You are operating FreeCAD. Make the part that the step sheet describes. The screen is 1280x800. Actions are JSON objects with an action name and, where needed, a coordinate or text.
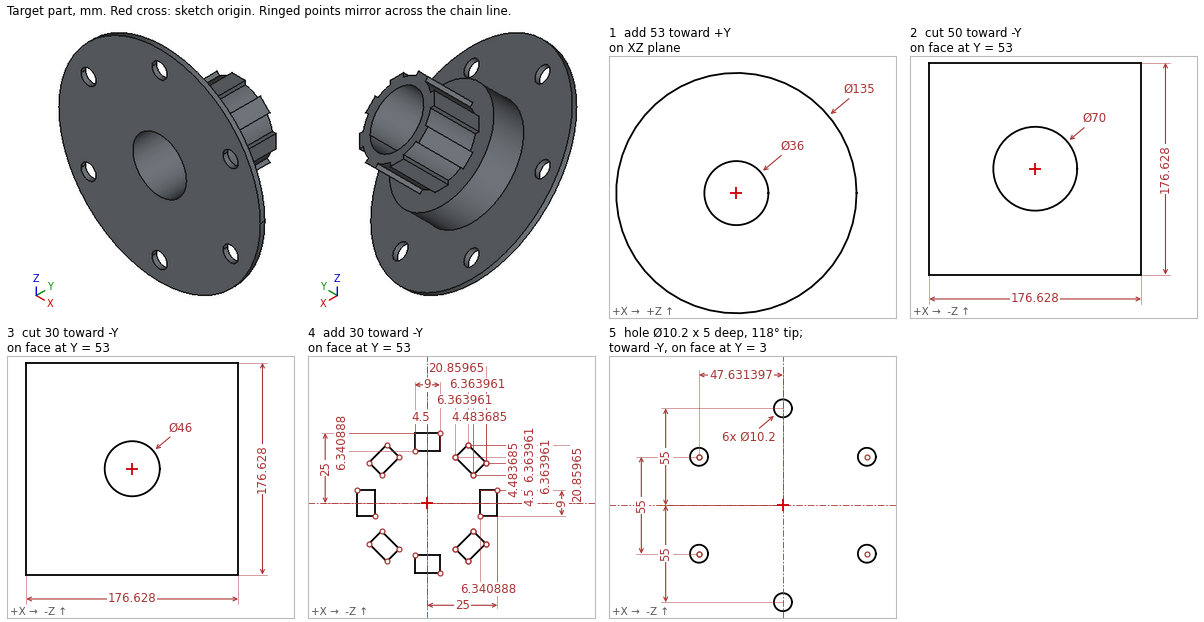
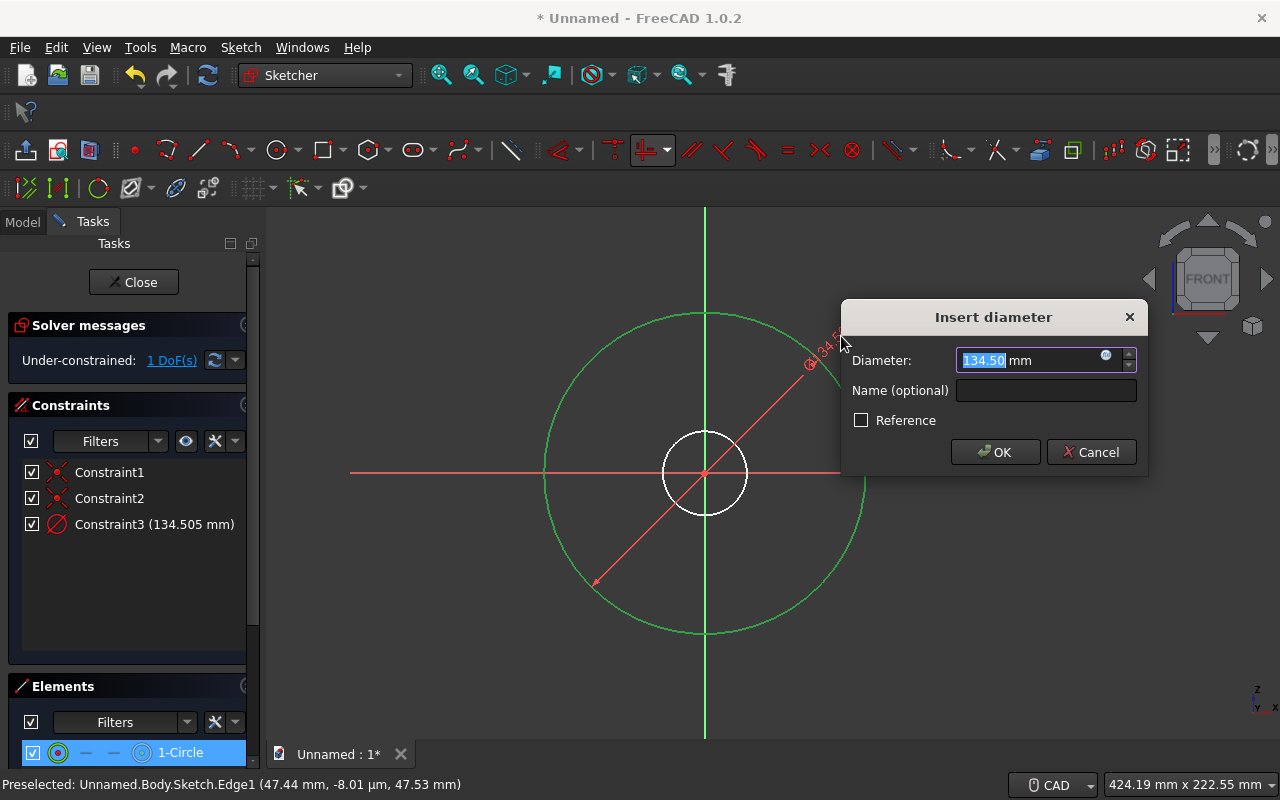
{"action": "type", "text": "135"}
{"action": "key", "text": "Return"}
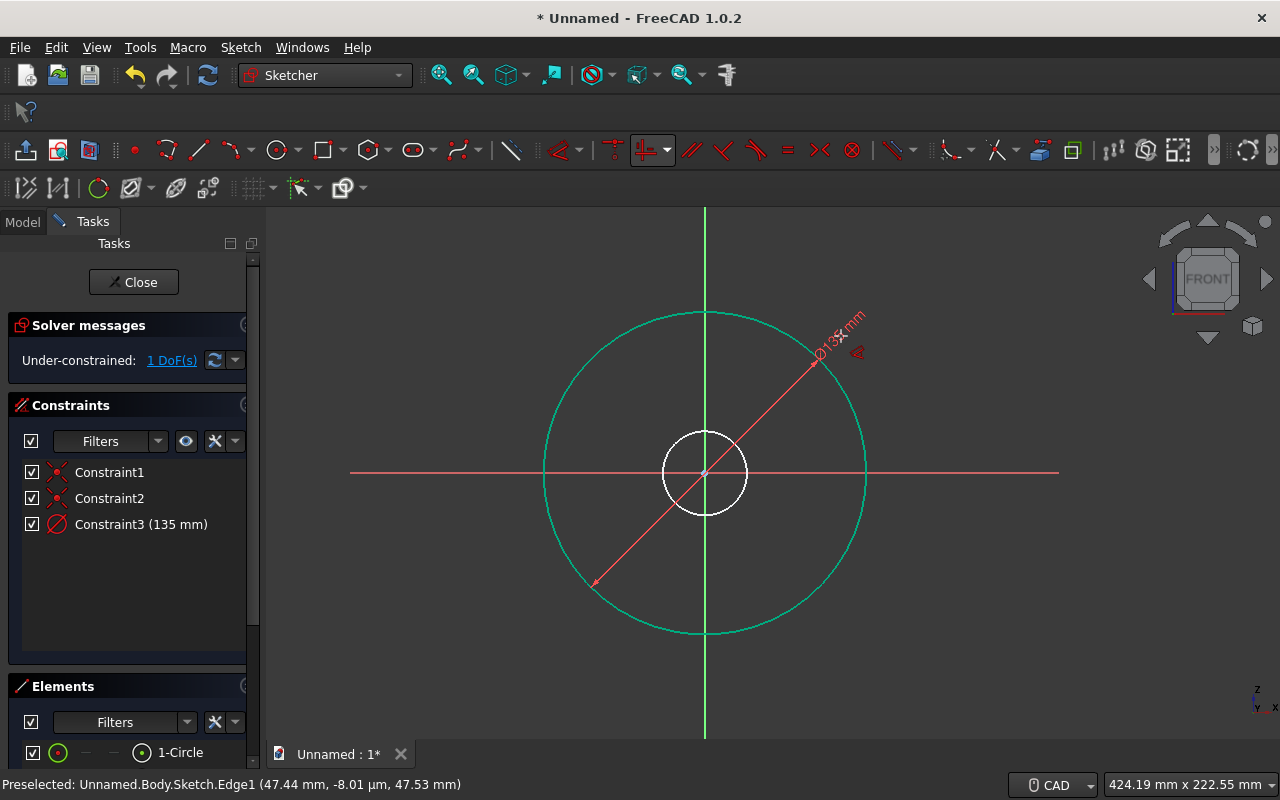
{"action": "left_click", "coordinate": [735, 444]}
{"action": "left_click", "coordinate": [758, 422]}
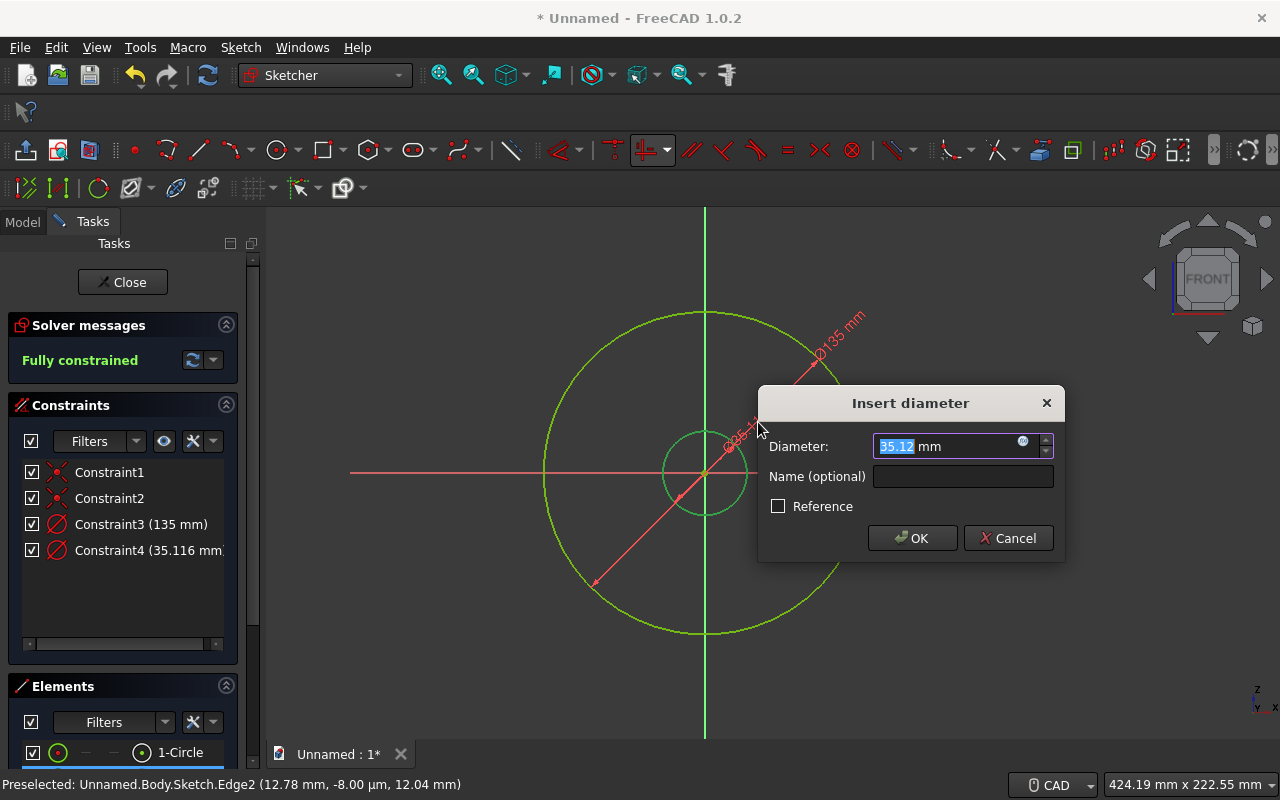
{"action": "type", "text": "36"}
{"action": "key", "text": "Return"}
{"action": "key", "text": "Escape"}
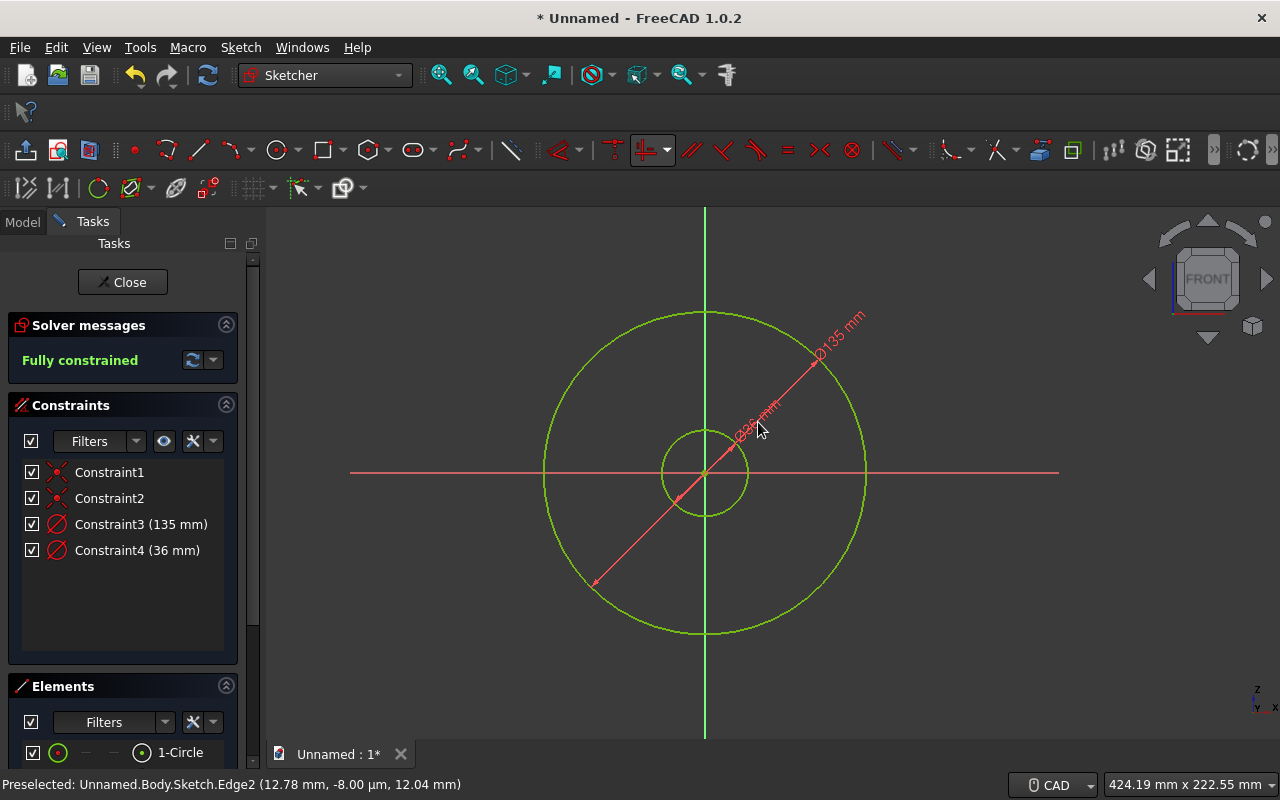
{"action": "left_click", "coordinate": [123, 282]}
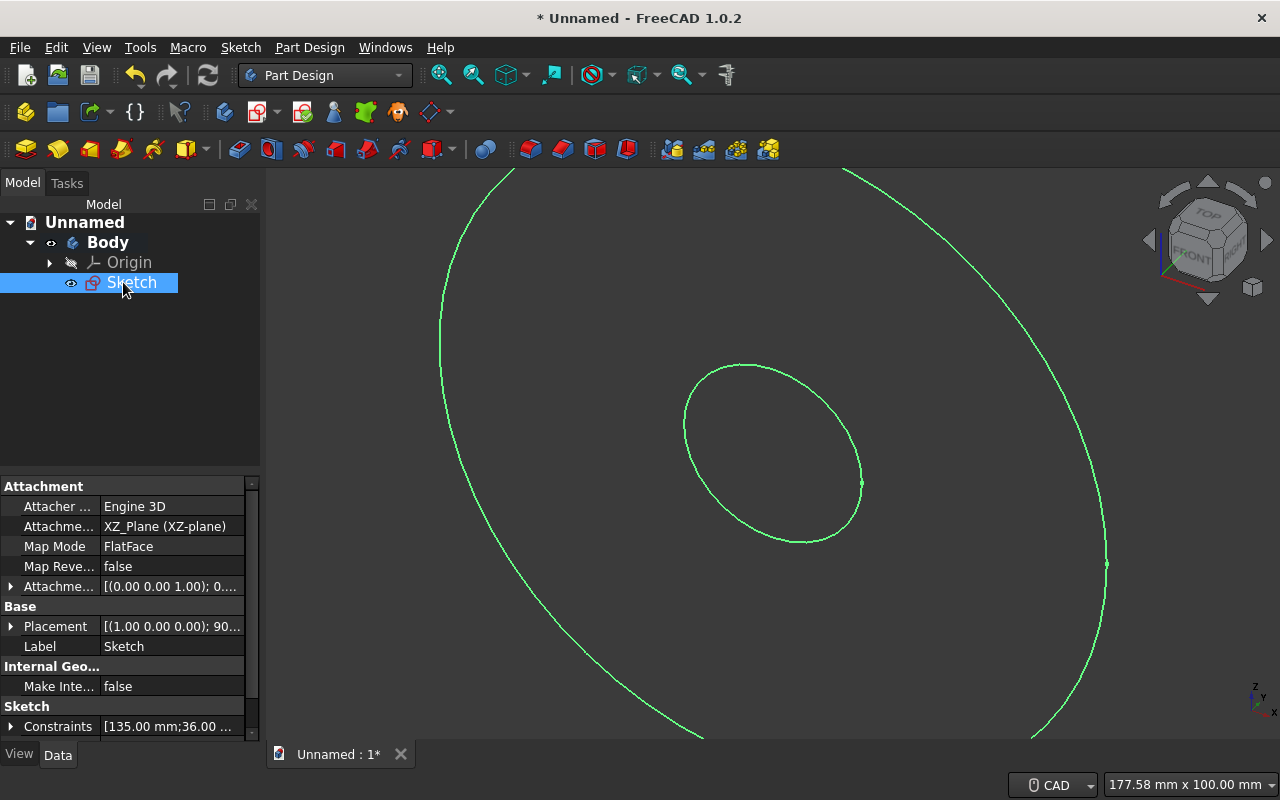
{"action": "left_click", "coordinate": [26, 150]}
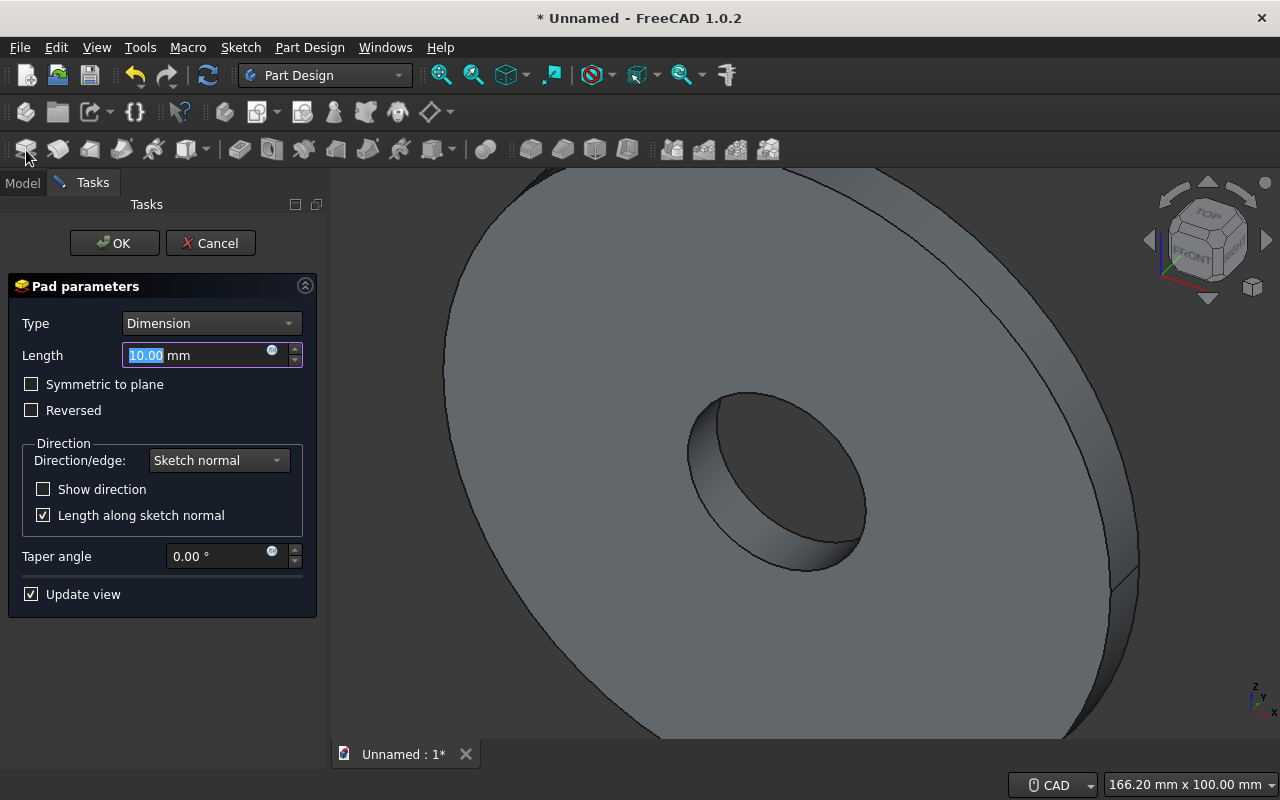
{"action": "type", "text": "53"}
{"action": "key", "text": "Tab"}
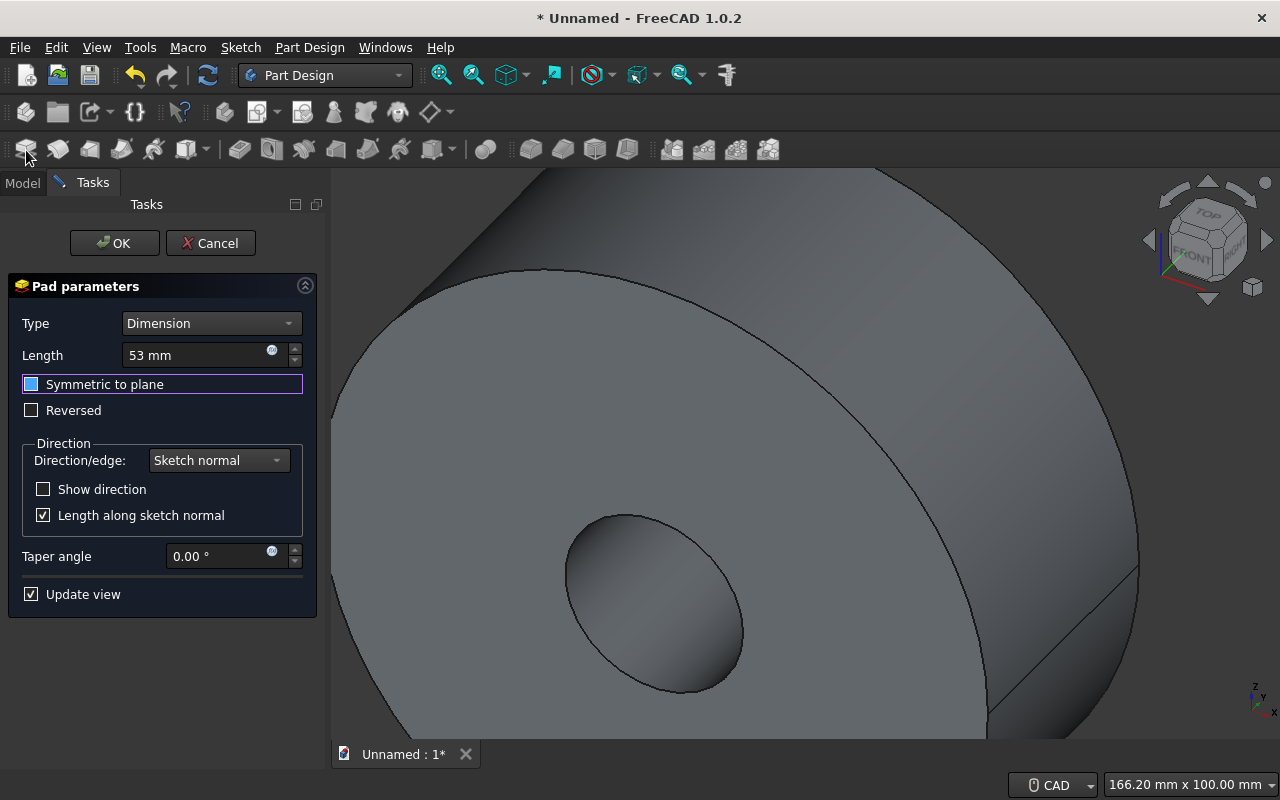
{"action": "left_click", "coordinate": [30, 410]}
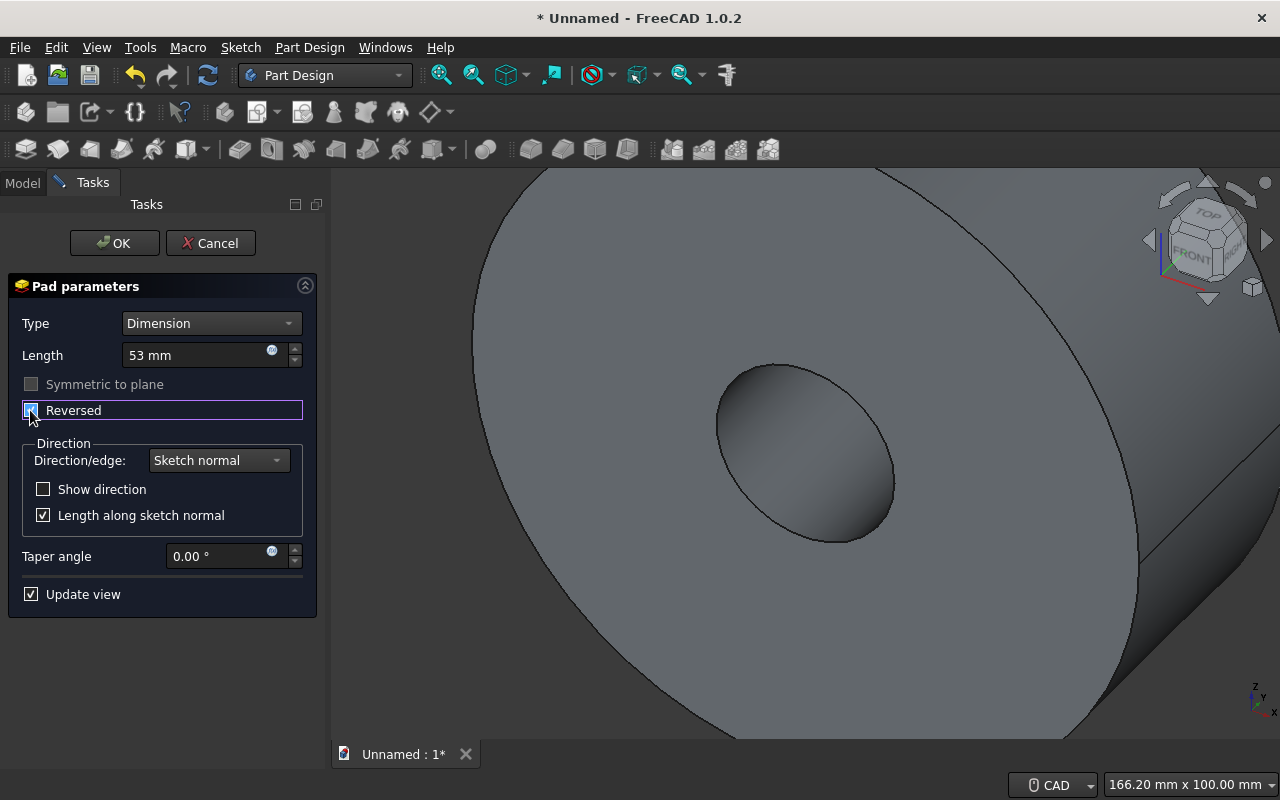
{"action": "left_click", "coordinate": [115, 243]}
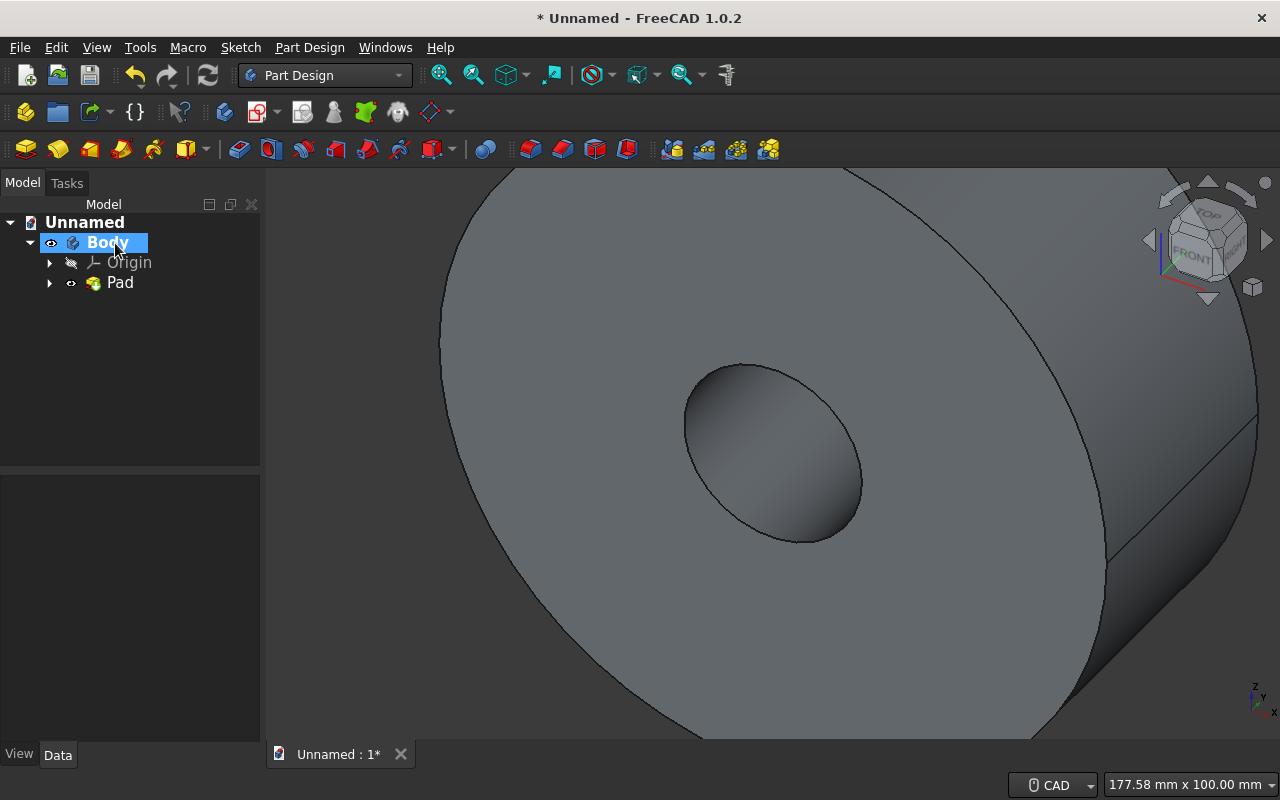
{"action": "left_click", "coordinate": [442, 76]}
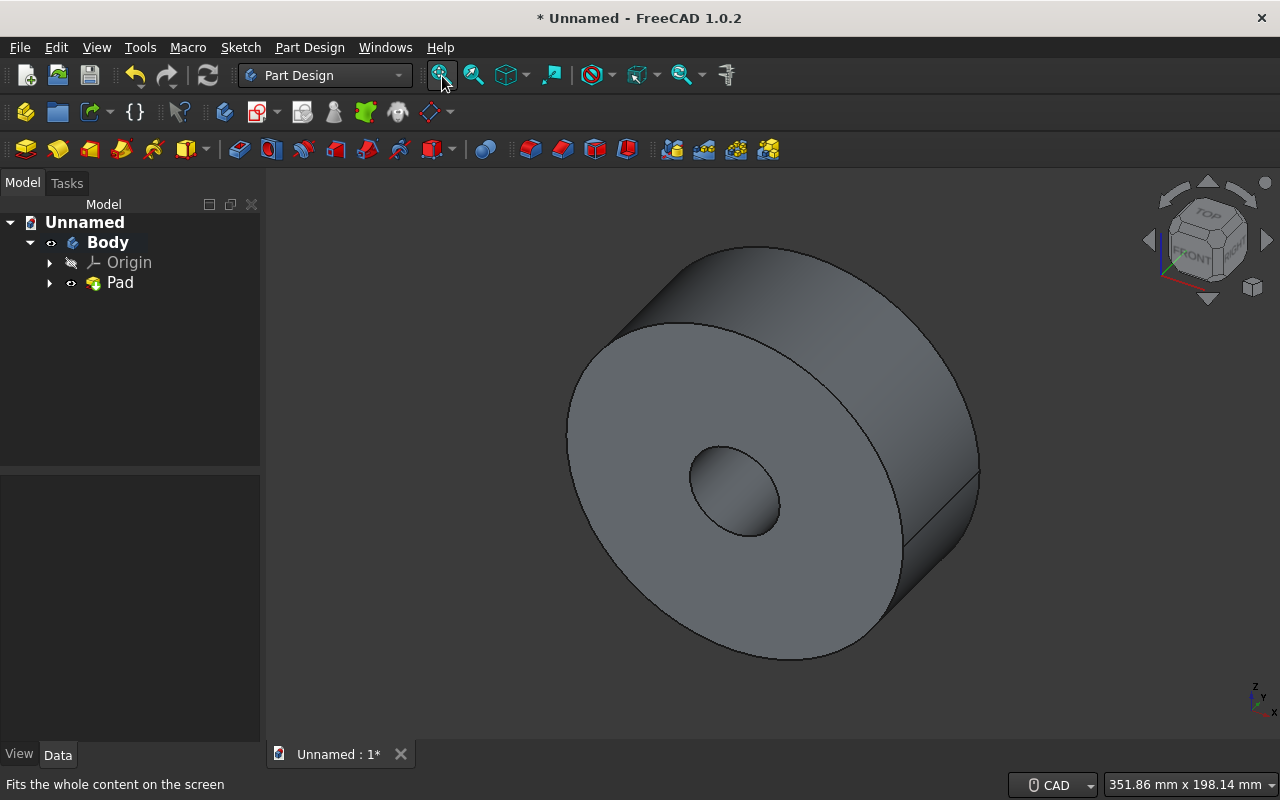
{"action": "key", "text": "4"}